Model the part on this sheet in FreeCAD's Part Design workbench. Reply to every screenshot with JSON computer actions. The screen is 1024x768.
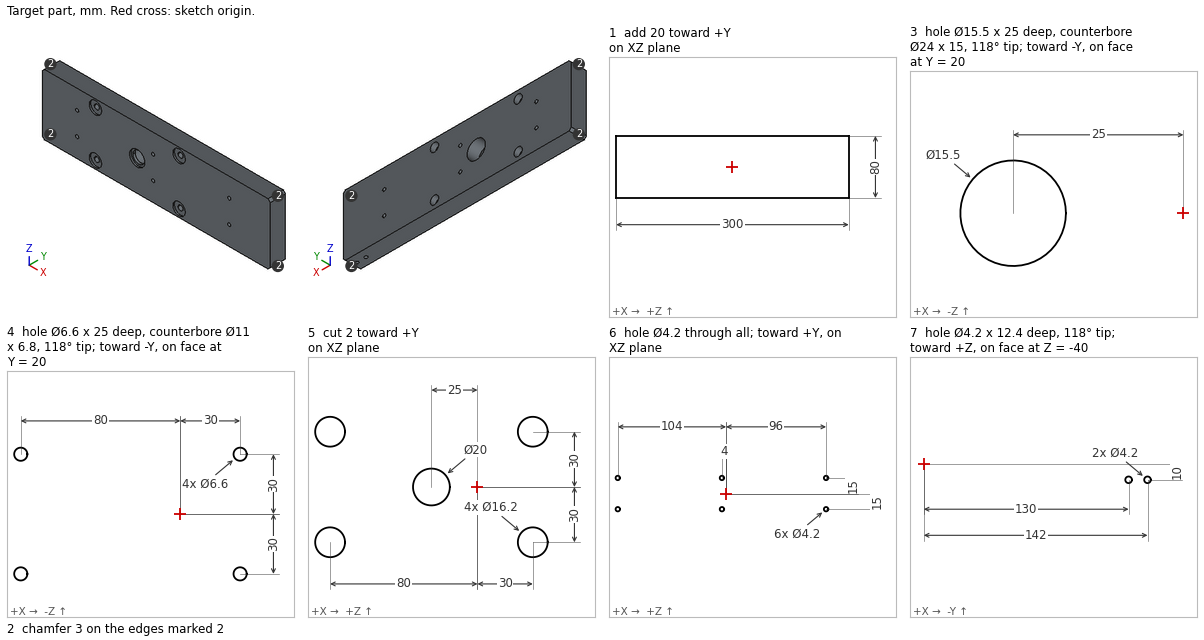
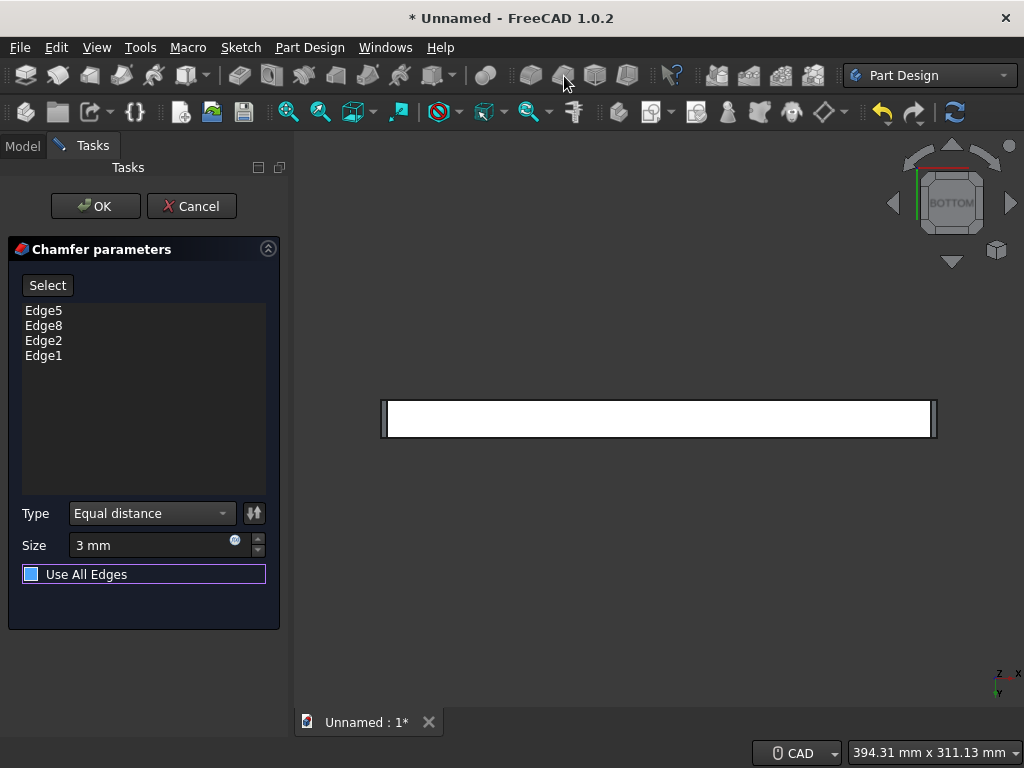
{"action": "left_click", "coordinate": [96, 206]}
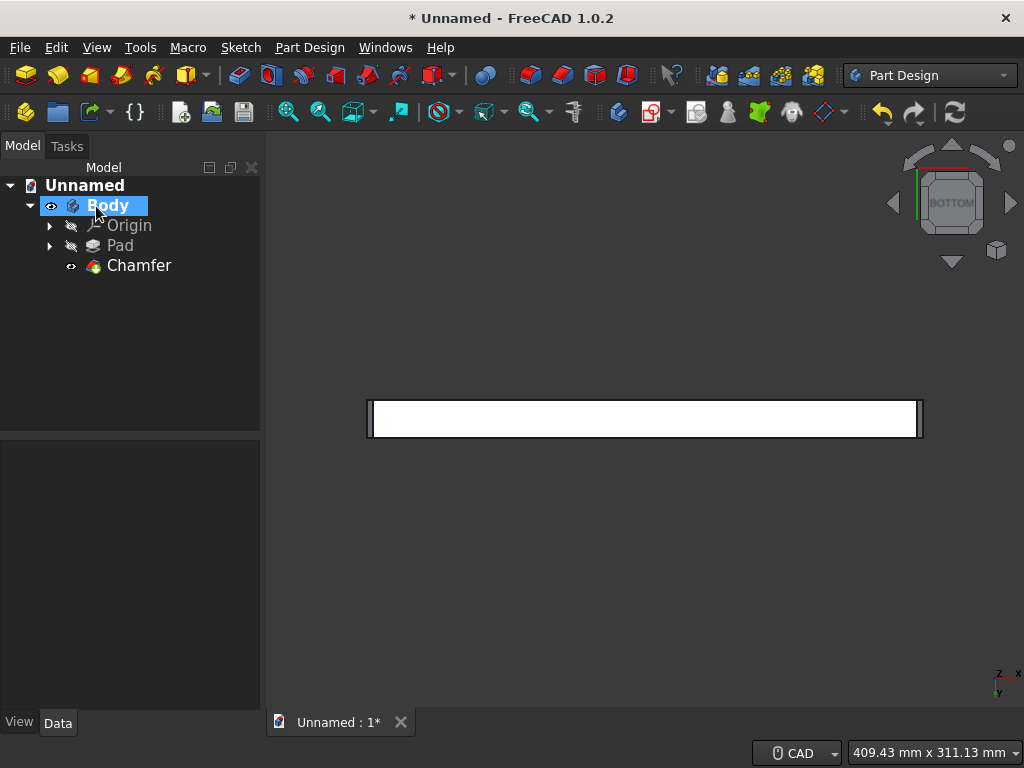
{"action": "key", "text": "4"}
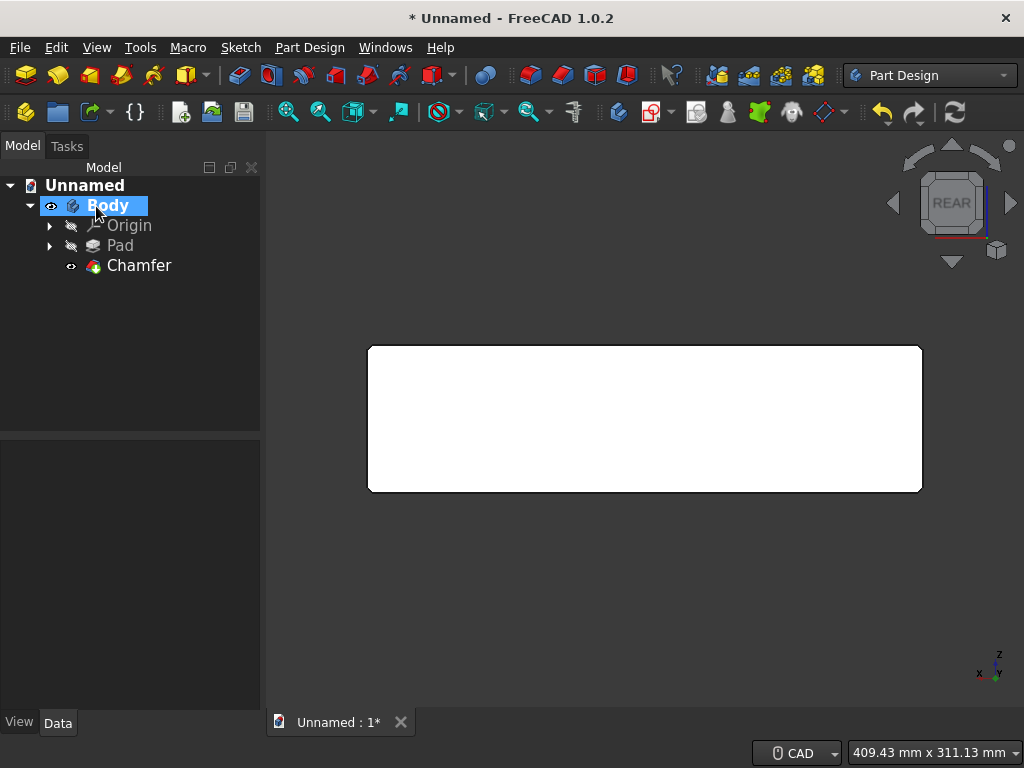
{"action": "left_click", "coordinate": [486, 418]}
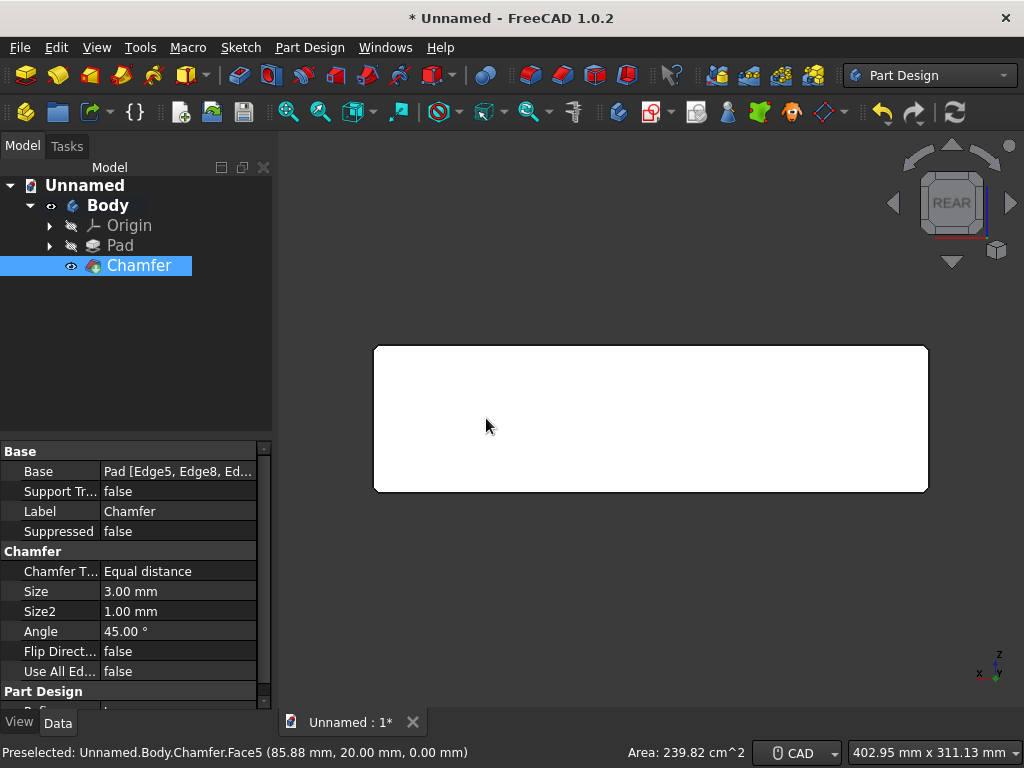
{"action": "left_click", "coordinate": [652, 112]}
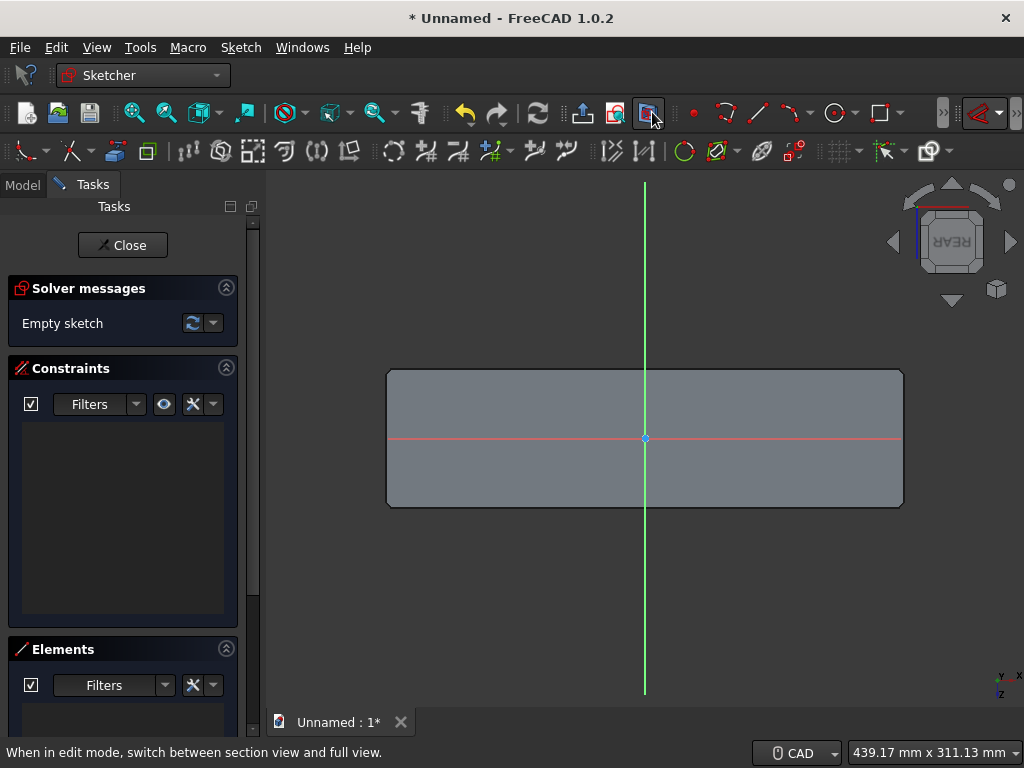
{"action": "scroll", "coordinate": [623, 439], "scroll_direction": "up", "scroll_amount": 10}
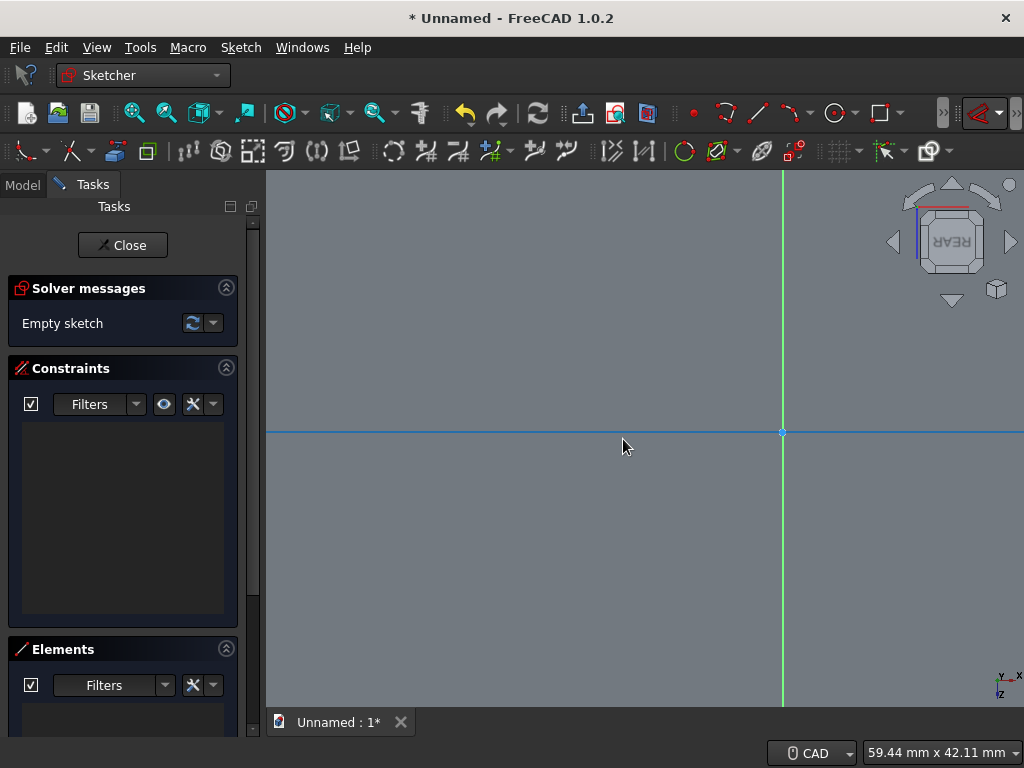
{"action": "left_click", "coordinate": [836, 114]}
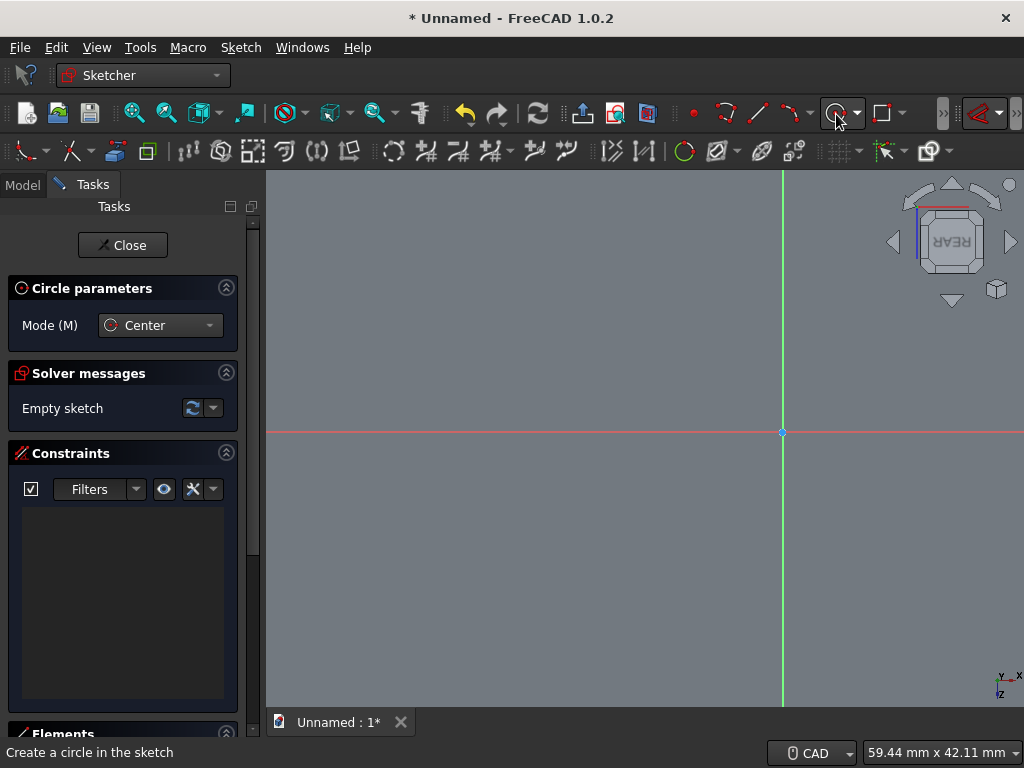
{"action": "left_click", "coordinate": [464, 432]}
{"action": "mouse_move", "coordinate": [534, 362]}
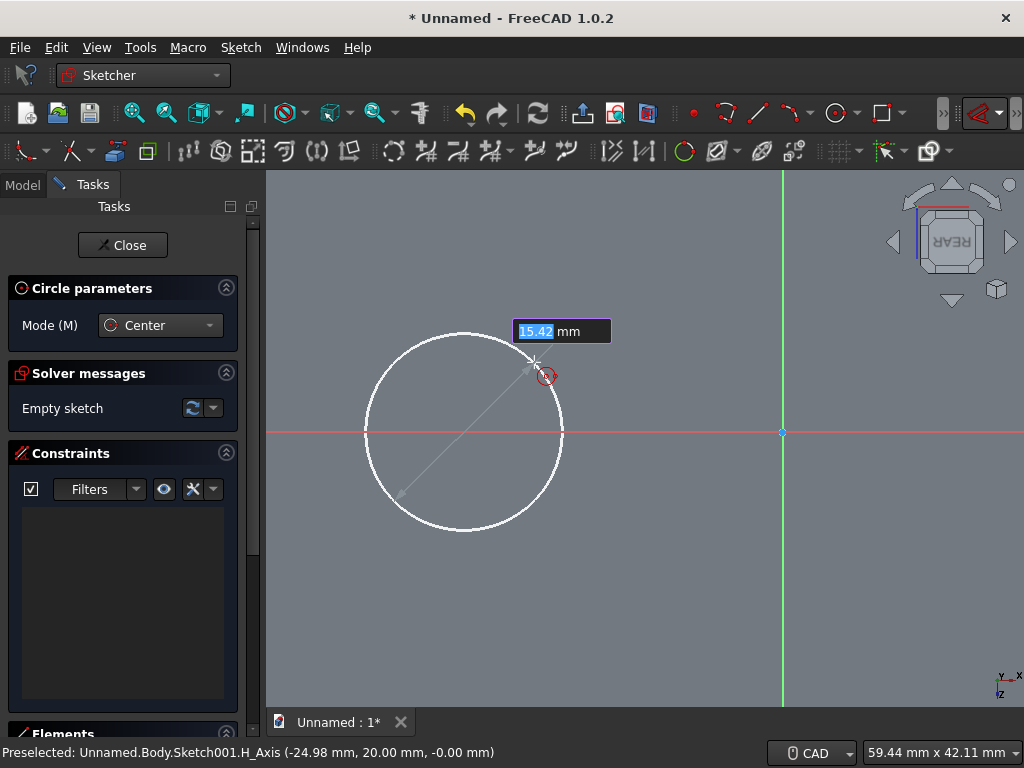
{"action": "type", "text": "15.5"}
{"action": "key", "text": "Return"}
{"action": "key", "text": "Escape"}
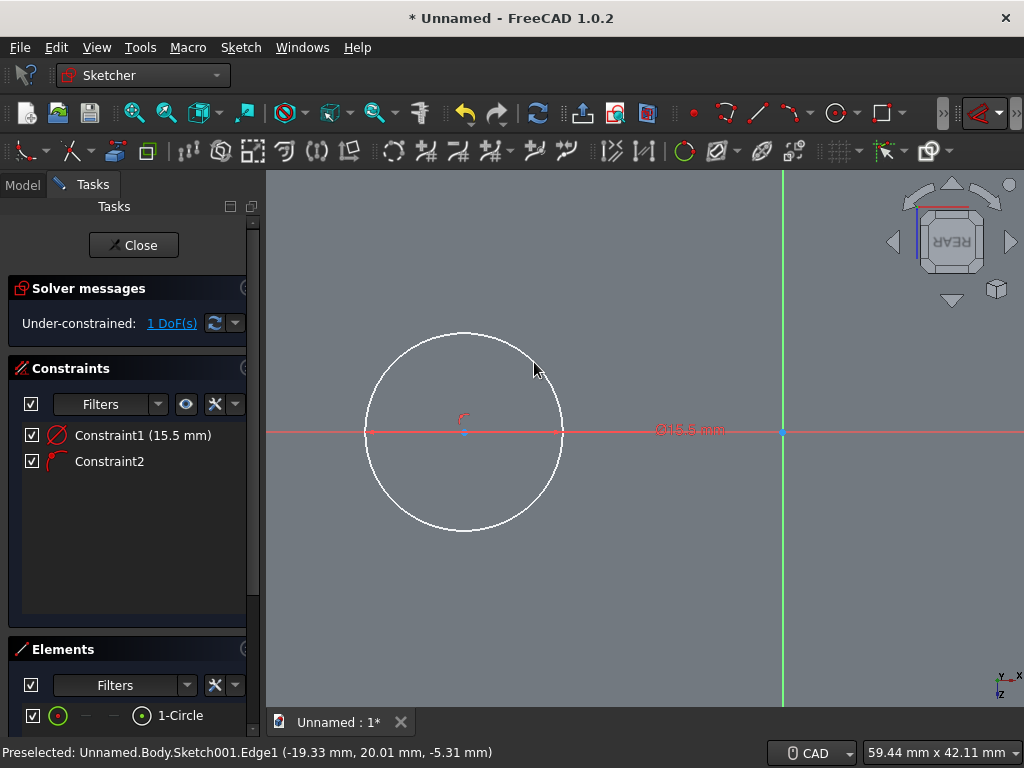
{"action": "left_click", "coordinate": [978, 114]}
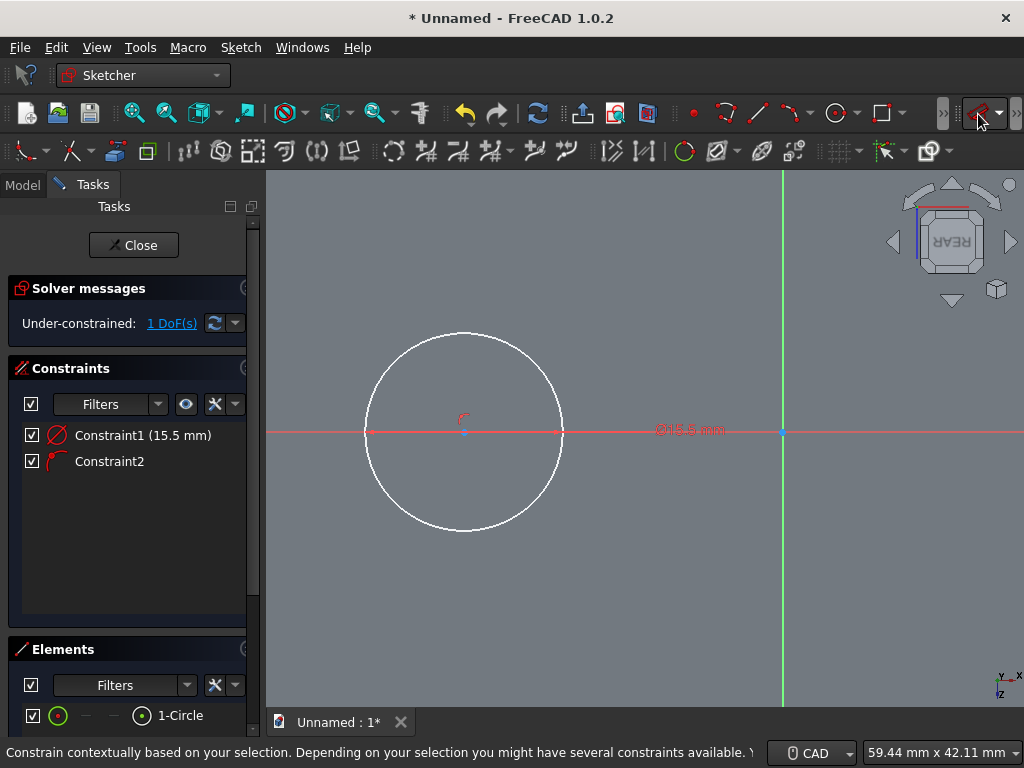
{"action": "left_click", "coordinate": [464, 432]}
{"action": "left_click", "coordinate": [623, 466]}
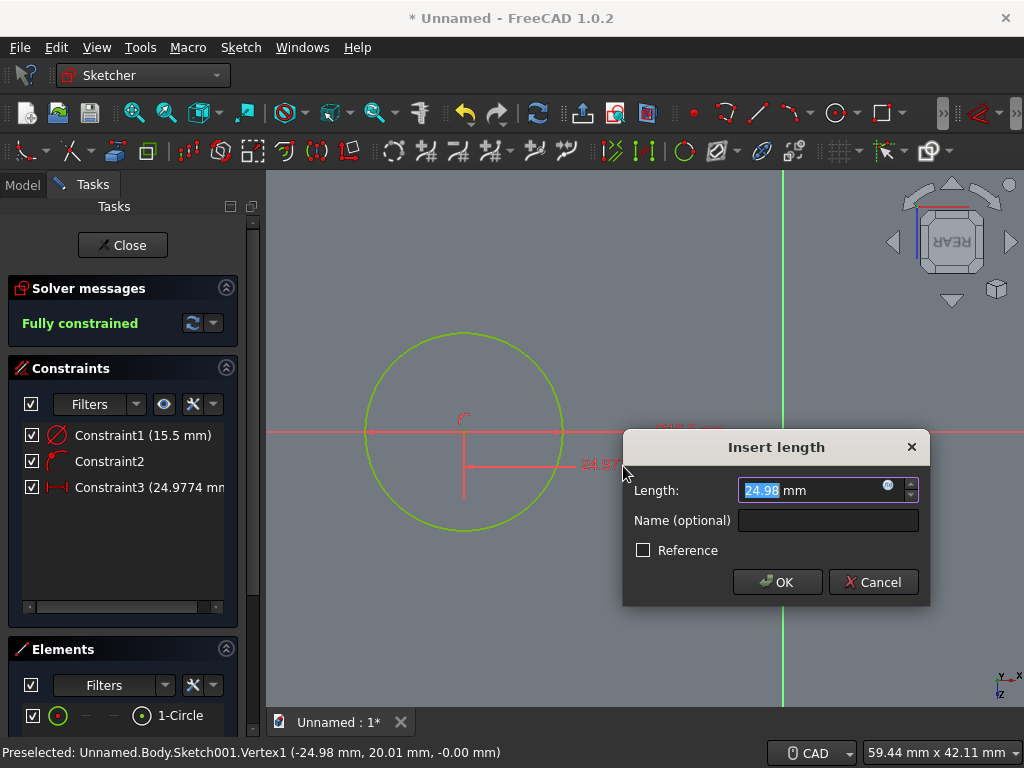
{"action": "type", "text": "25"}
{"action": "key", "text": "Return"}
{"action": "key", "text": "Escape"}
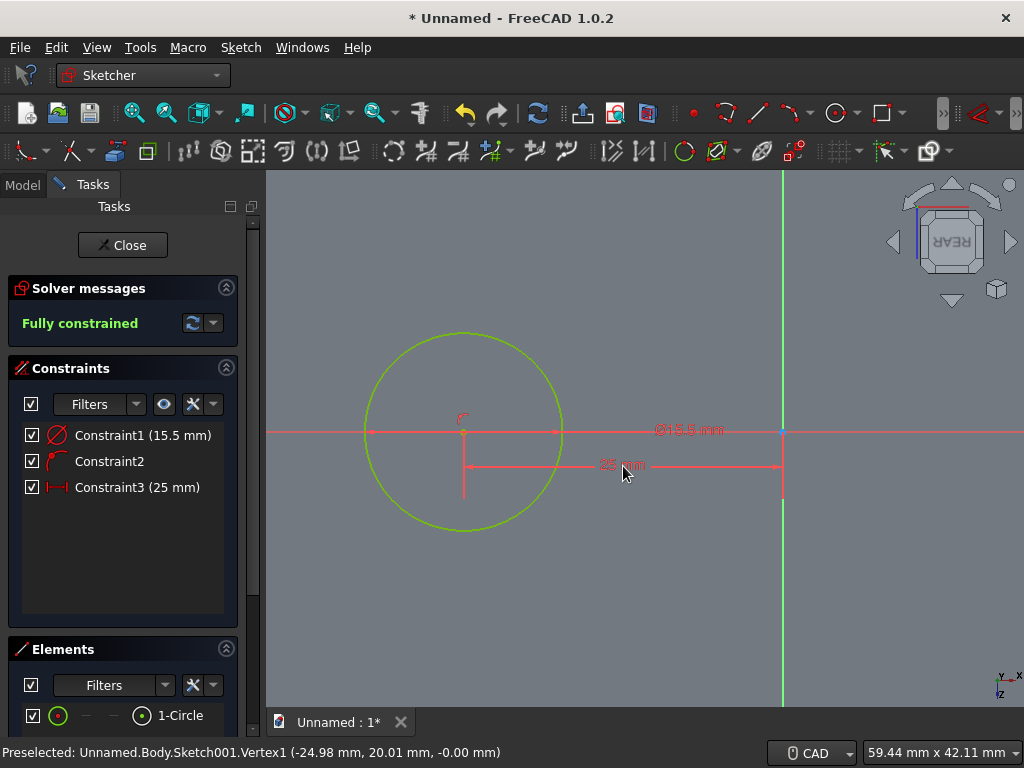
{"action": "left_click", "coordinate": [123, 245]}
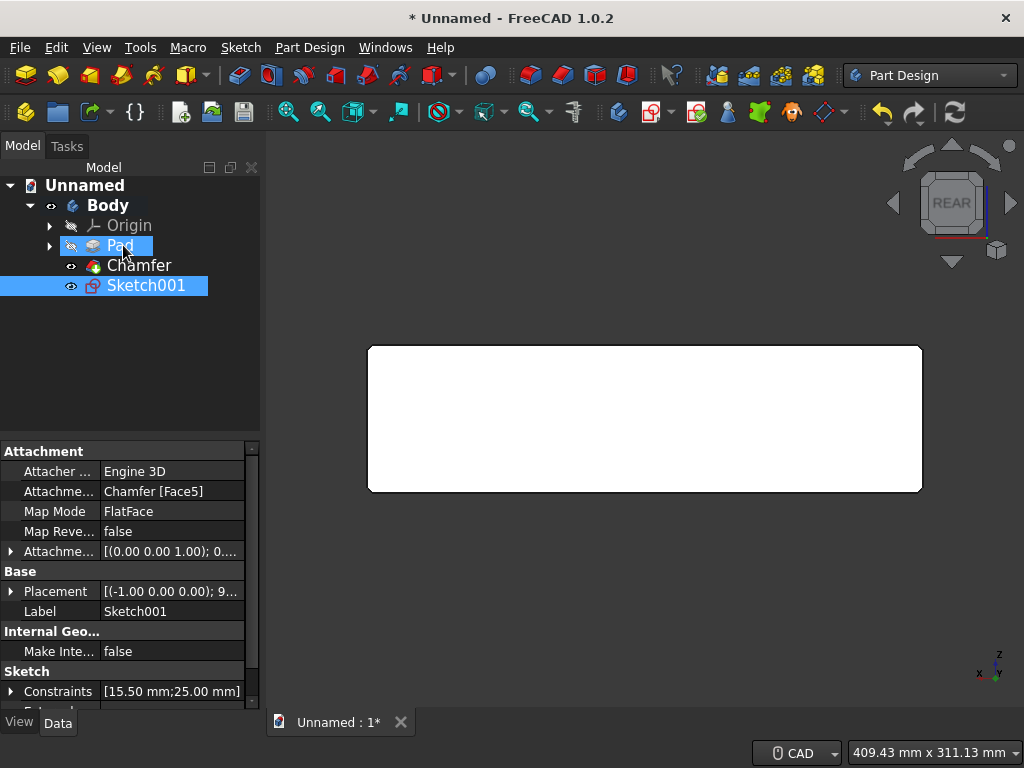
{"action": "left_click", "coordinate": [272, 76]}